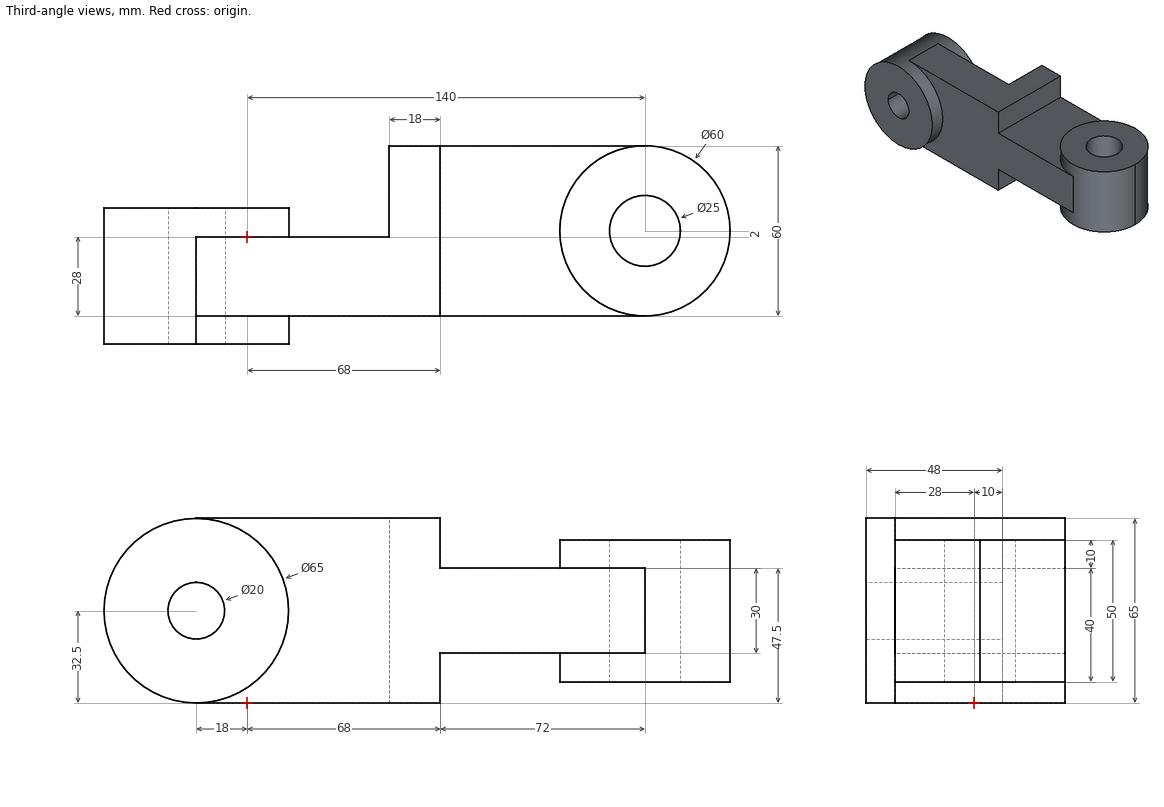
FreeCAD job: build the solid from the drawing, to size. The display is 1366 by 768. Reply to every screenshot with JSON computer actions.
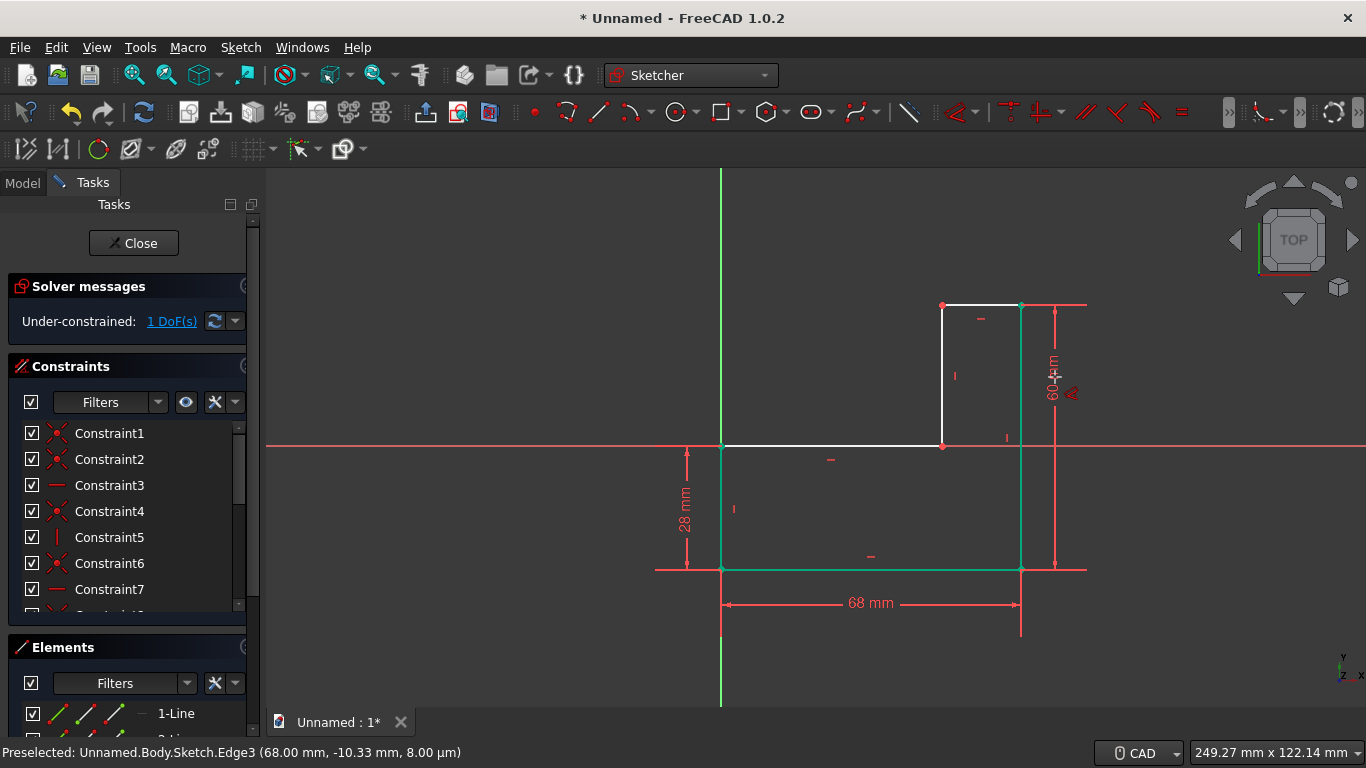
{"action": "left_click", "coordinate": [998, 305]}
{"action": "left_click", "coordinate": [982, 271]}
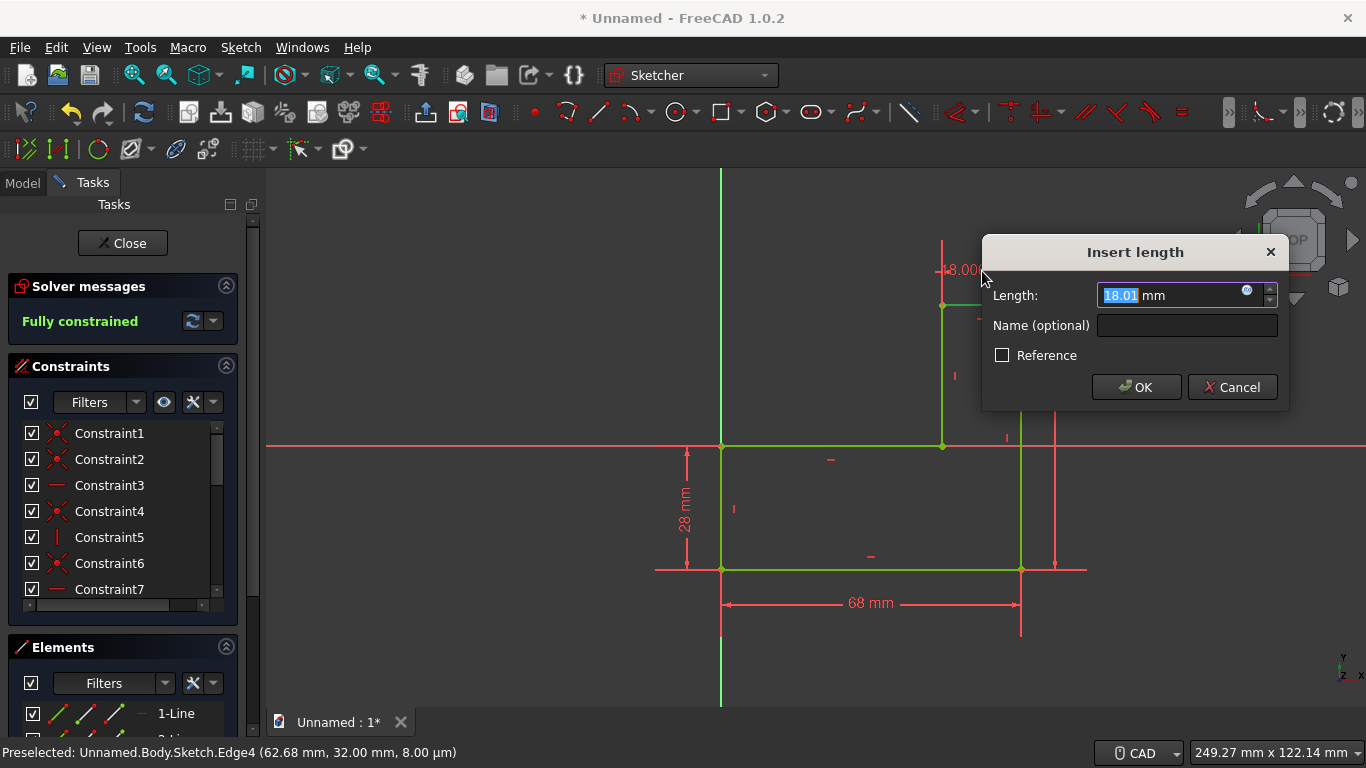
{"action": "type", "text": "18"}
{"action": "key", "text": "Return"}
{"action": "key", "text": "Escape"}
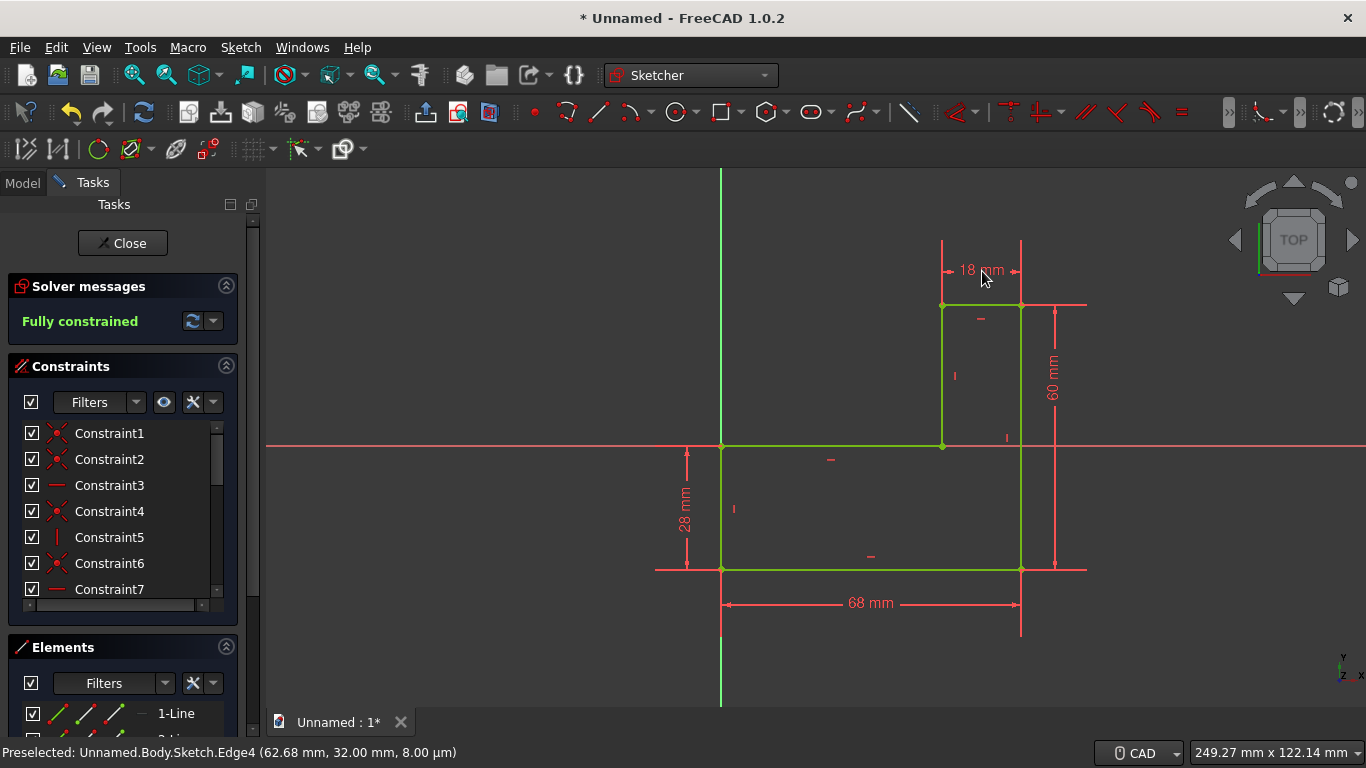
{"action": "left_click", "coordinate": [123, 243]}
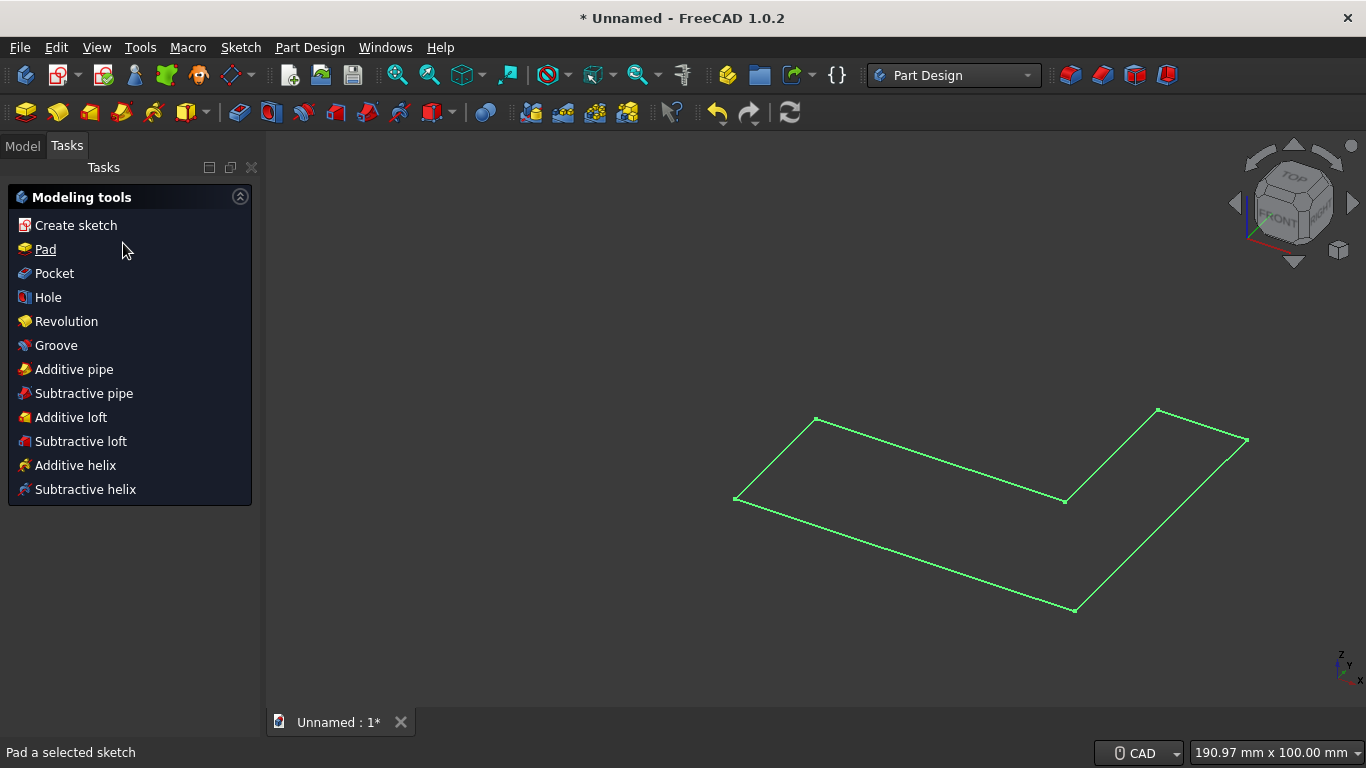
{"action": "left_click", "coordinate": [26, 112]}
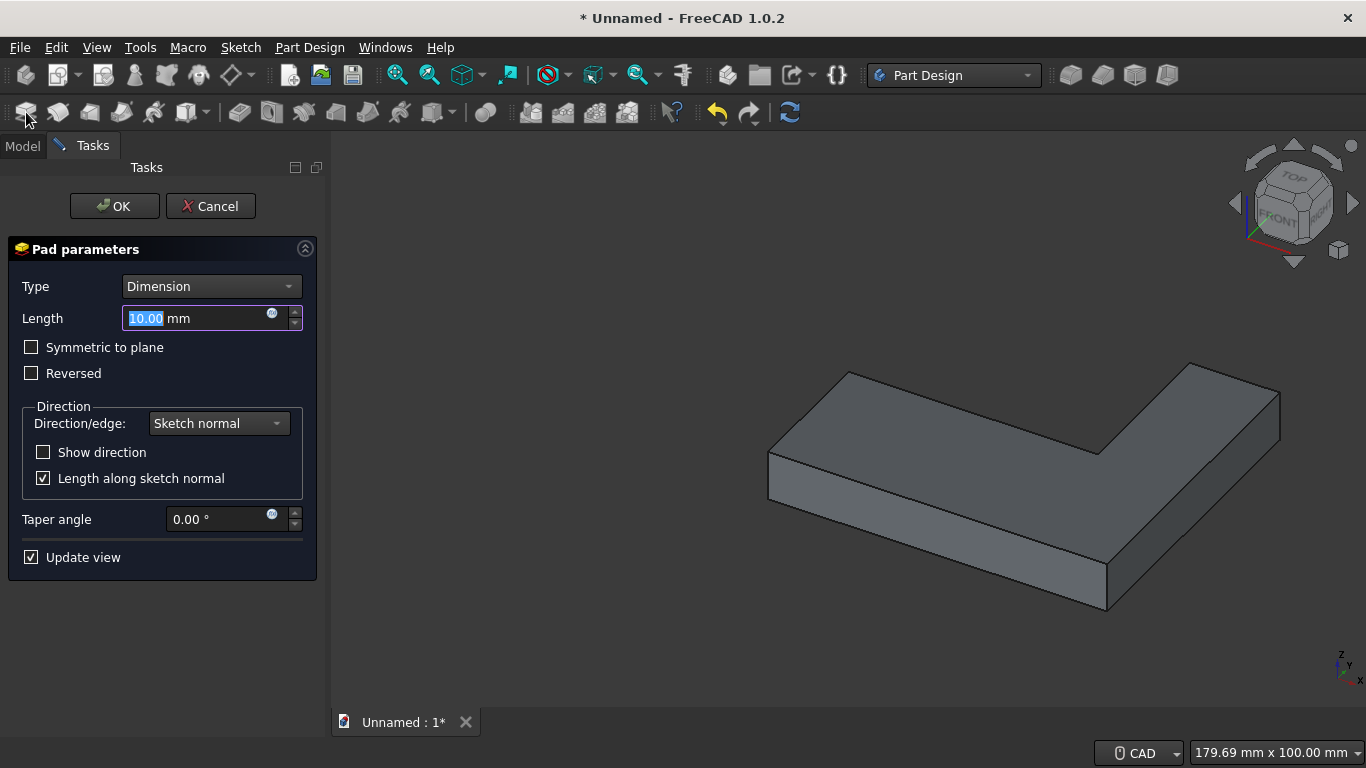
{"action": "type", "text": "65"}
{"action": "key", "text": "Tab"}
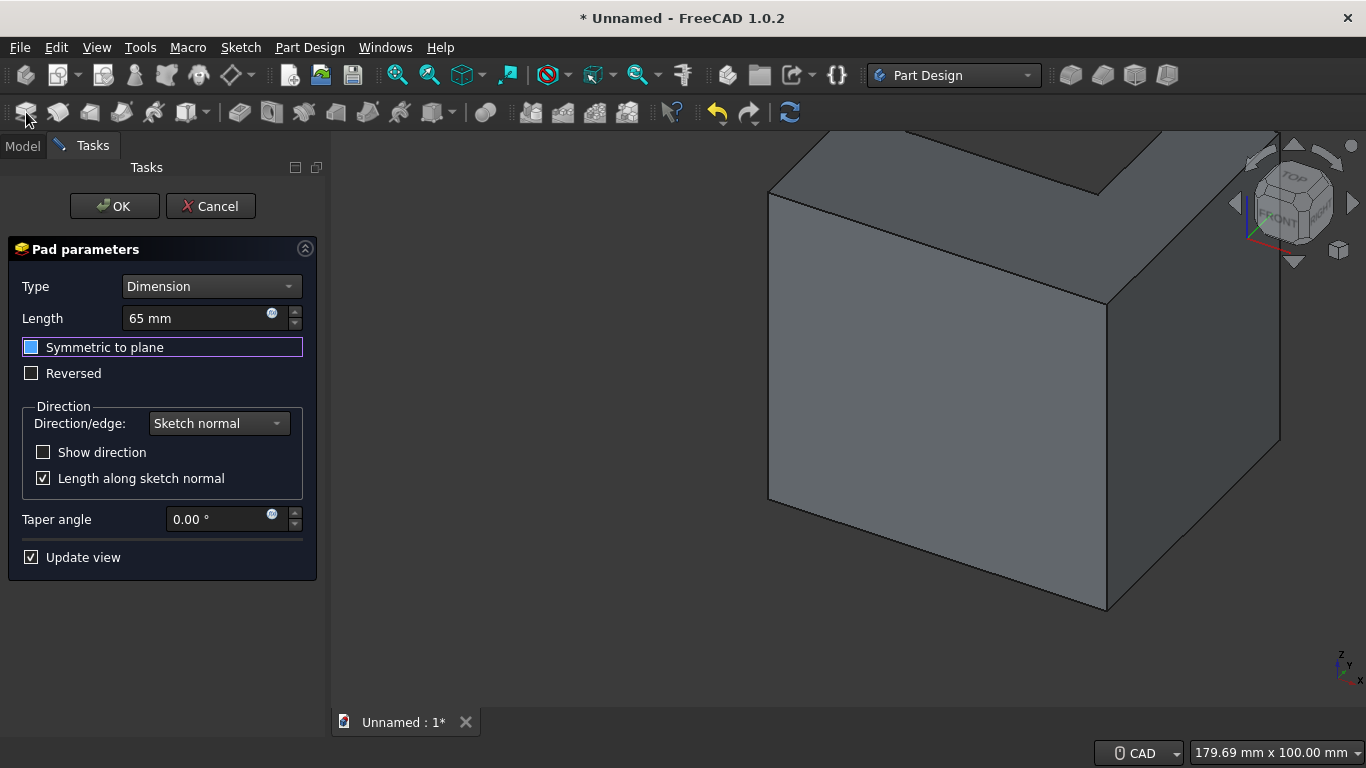
{"action": "left_click", "coordinate": [115, 206]}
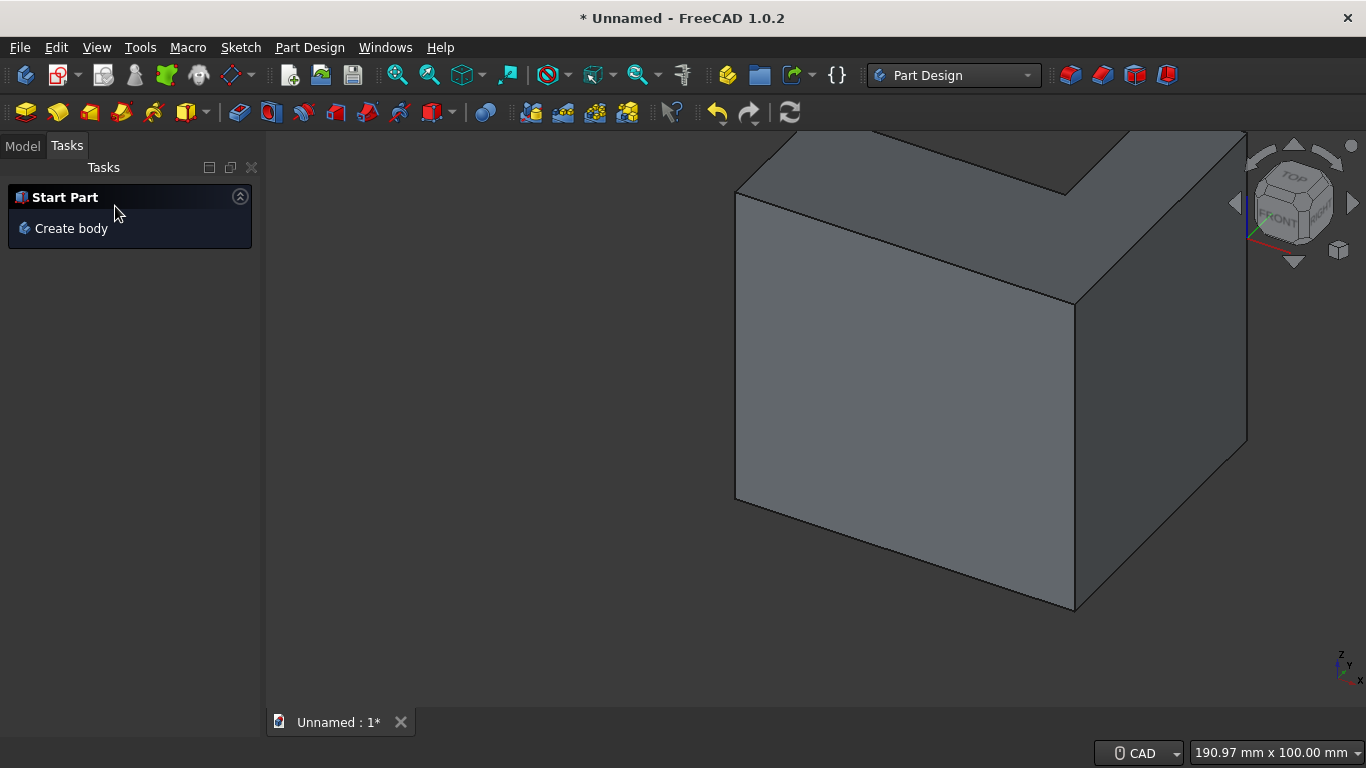
{"action": "key", "text": "v f"}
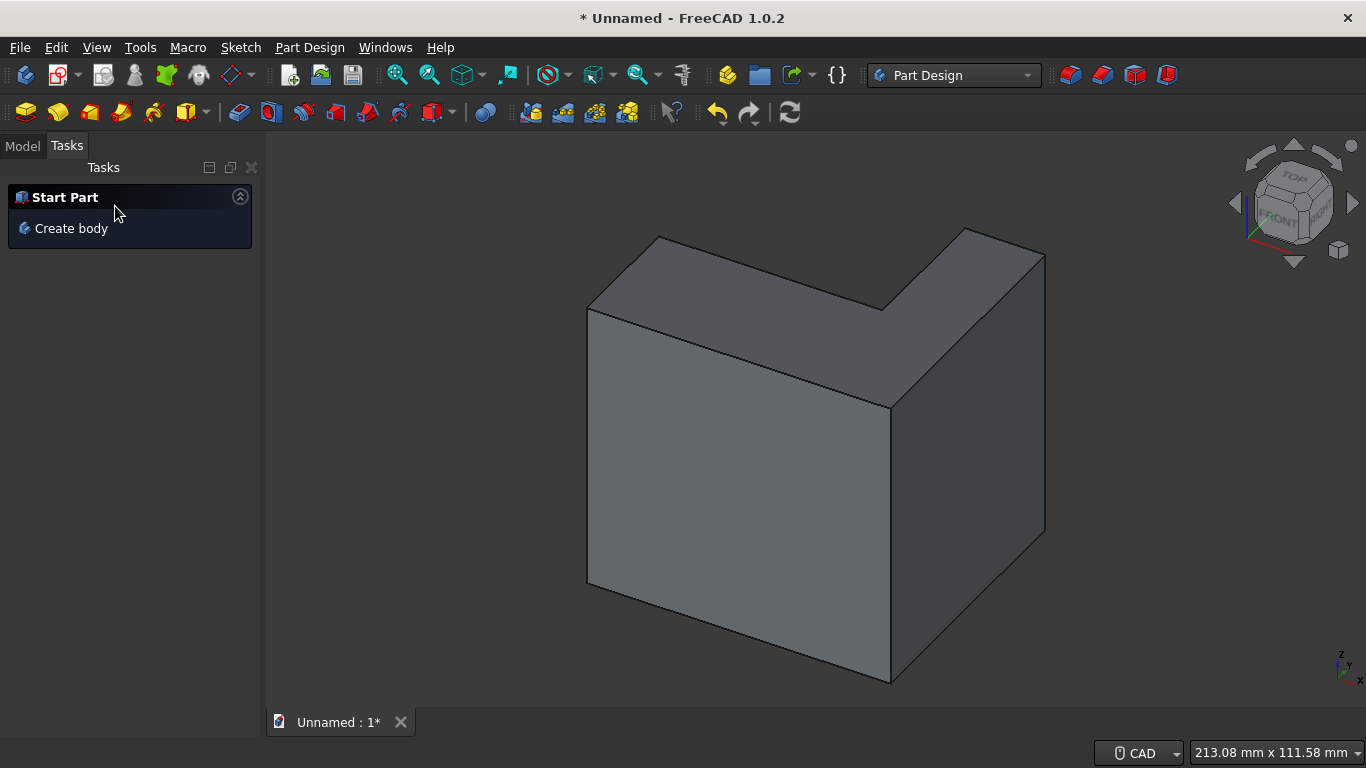
{"action": "left_click", "coordinate": [58, 76]}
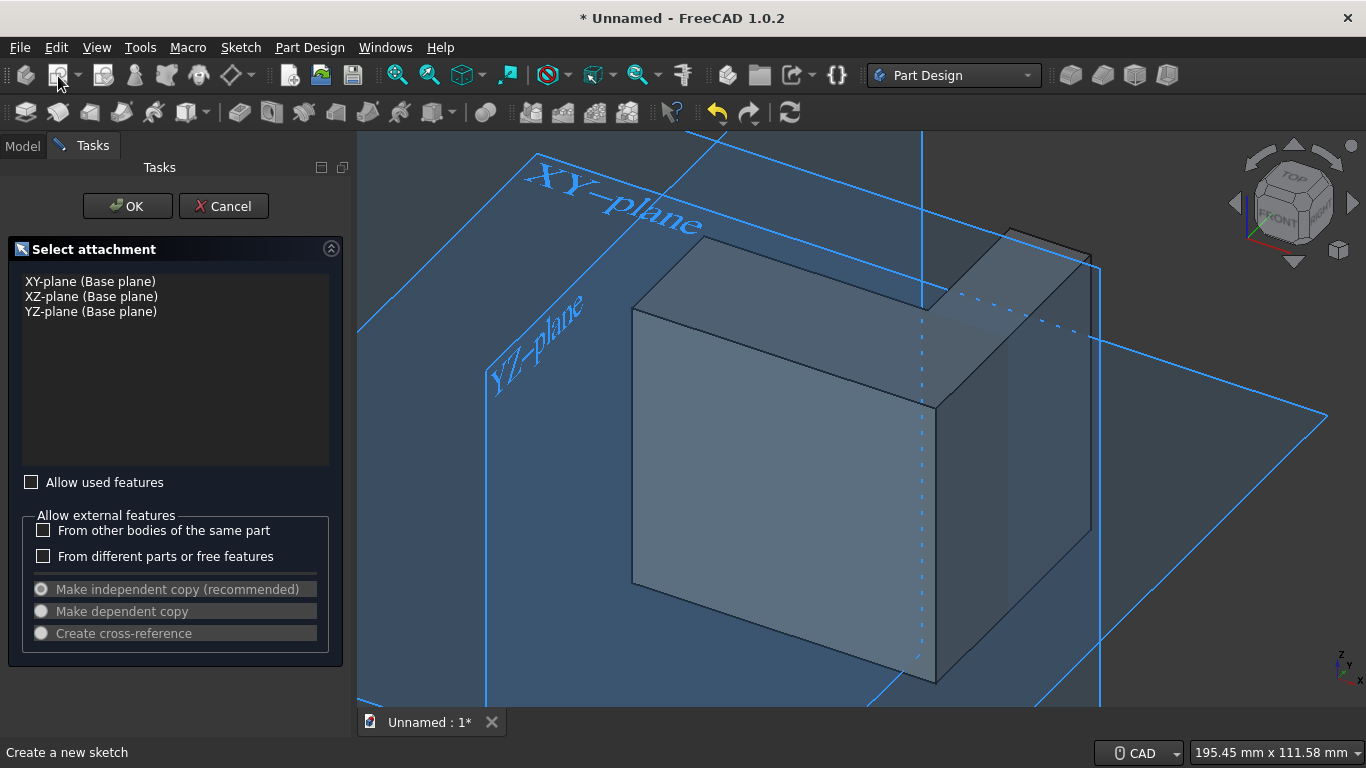
{"action": "left_click", "coordinate": [82, 312]}